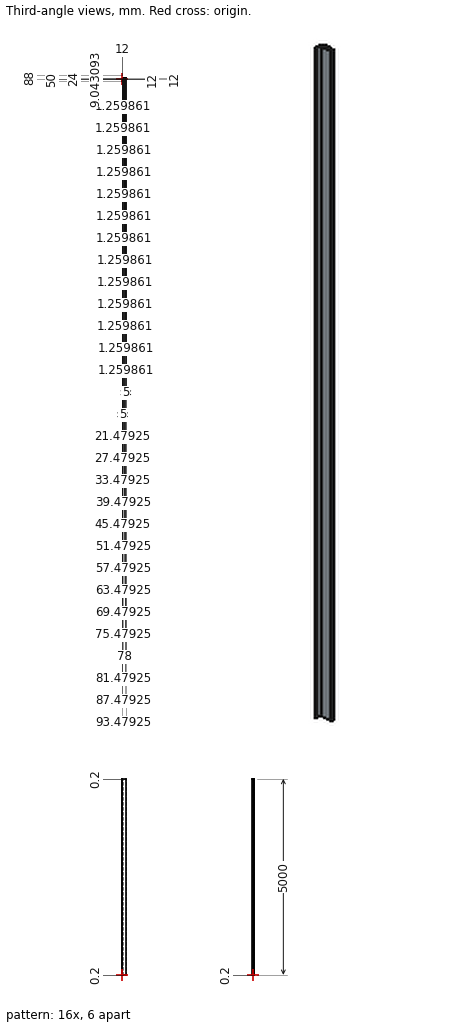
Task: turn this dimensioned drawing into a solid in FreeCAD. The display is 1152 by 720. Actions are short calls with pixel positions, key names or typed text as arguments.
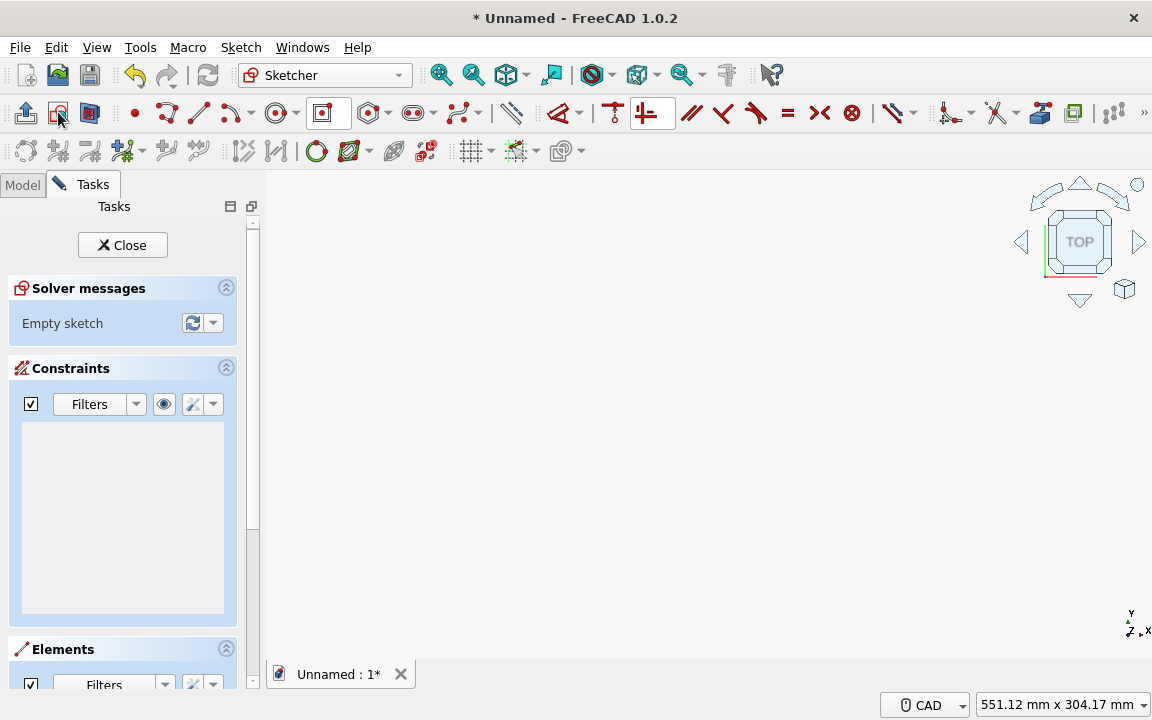
scroll(640, 414, down, 5)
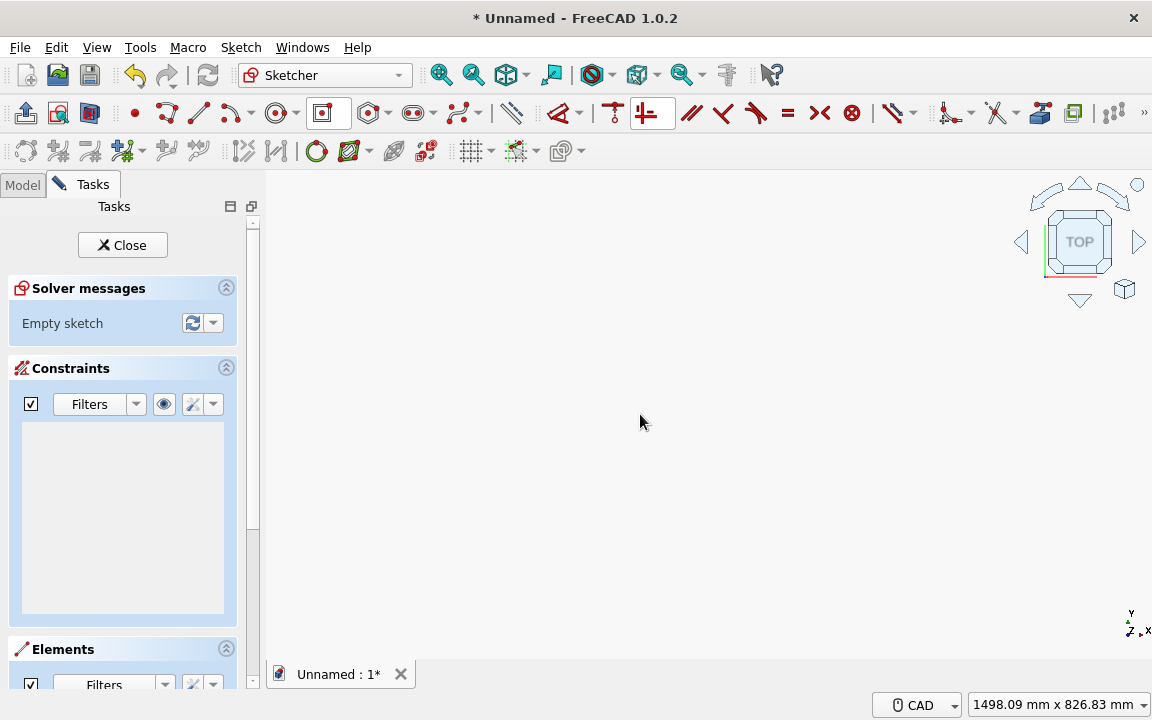
scroll(640, 414, down, 5)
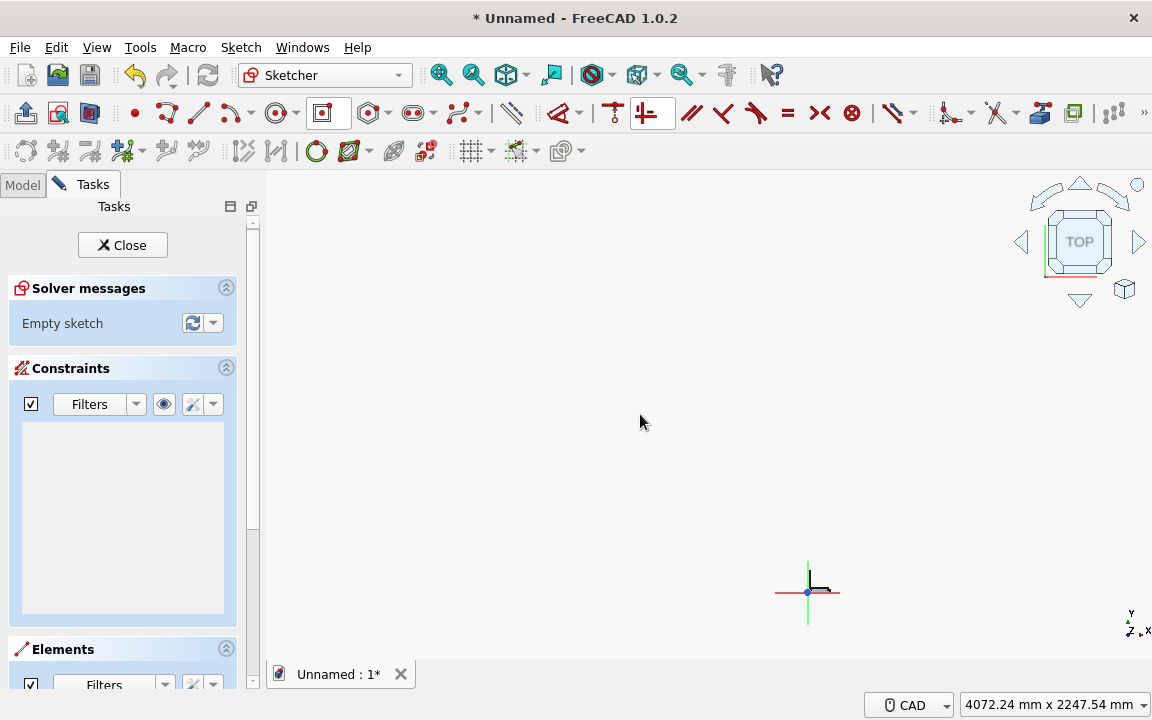
scroll(822, 598, up, 15)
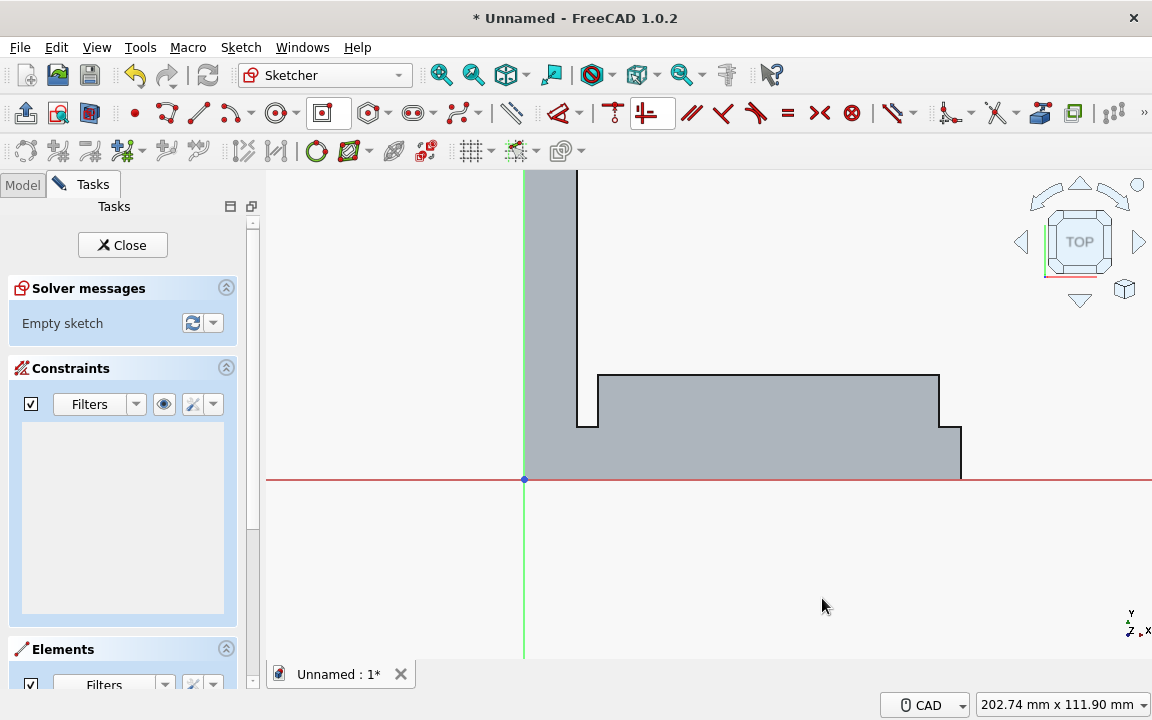
scroll(618, 392, up, 10)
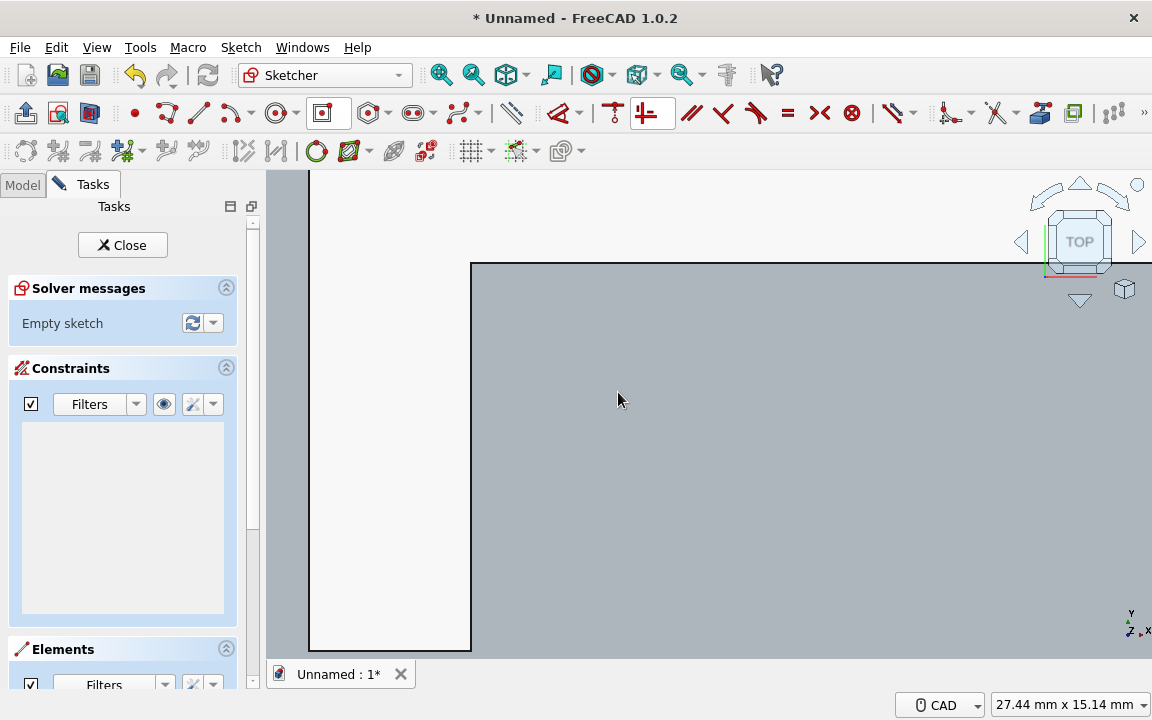
click(346, 114)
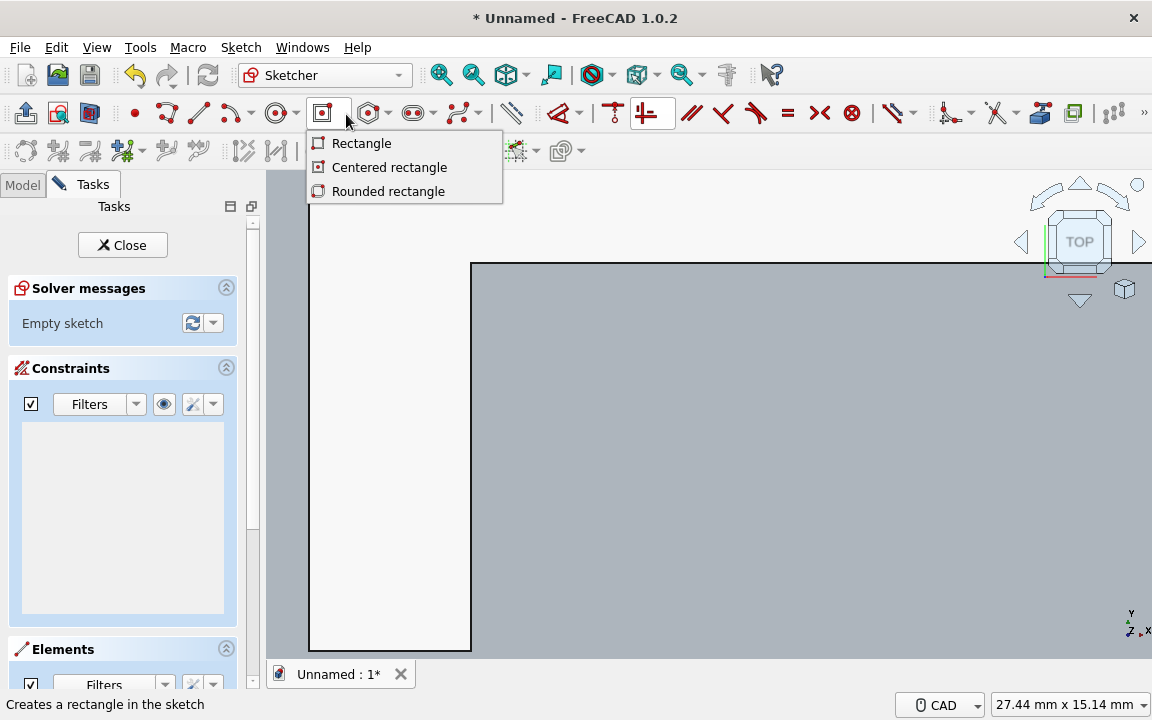
click(404, 143)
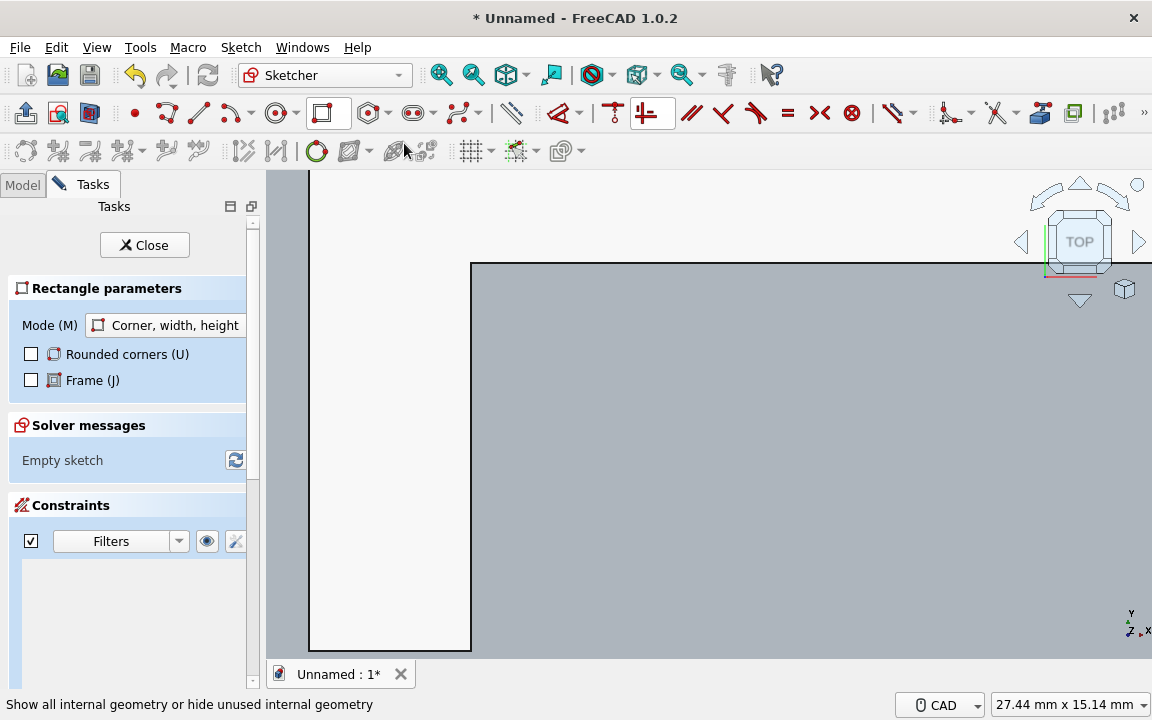
click(615, 263)
click(656, 555)
key(Escape)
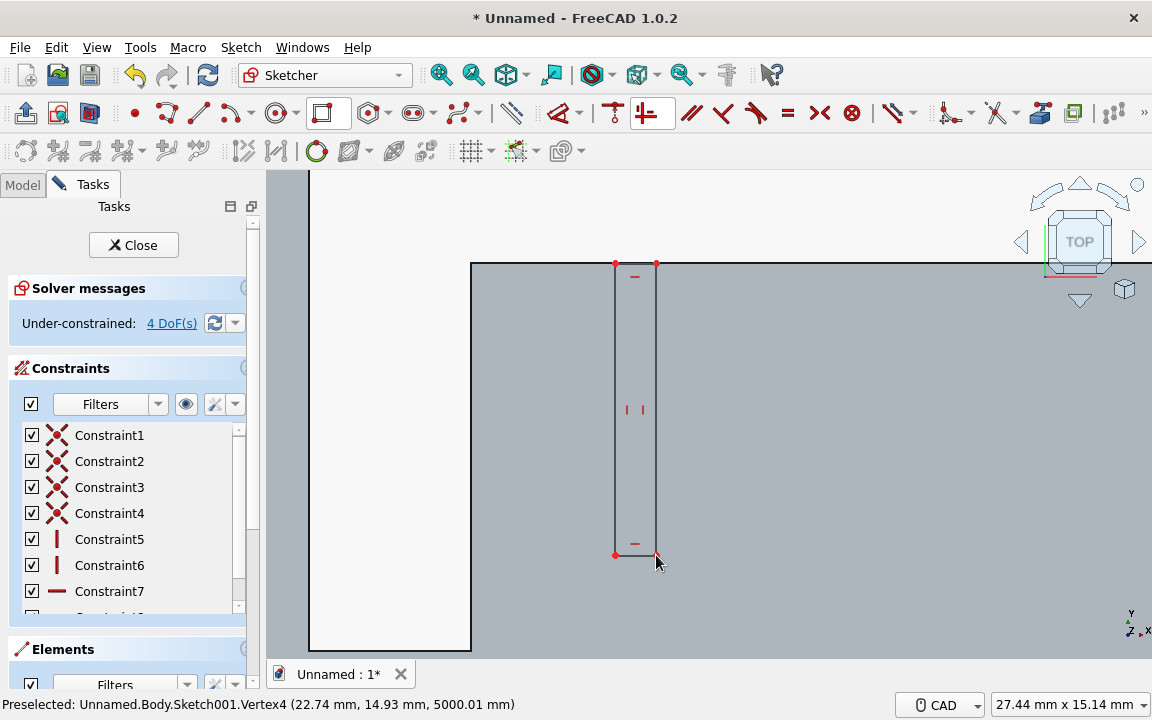
click(558, 114)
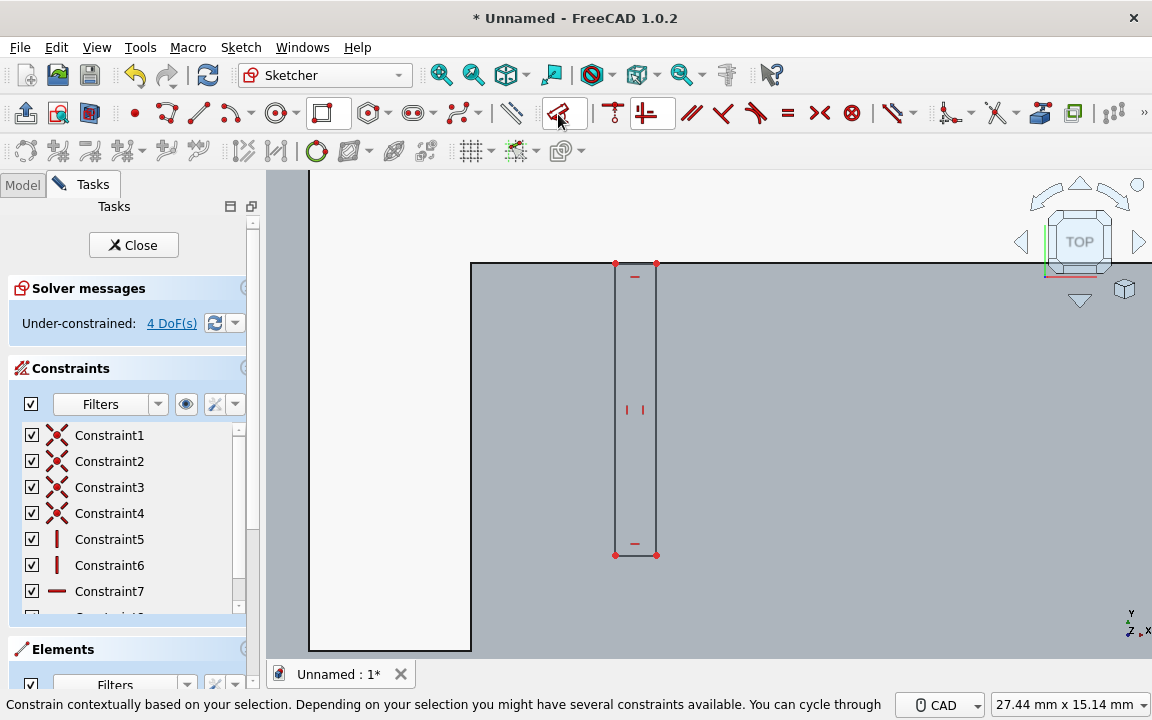
click(615, 264)
click(649, 576)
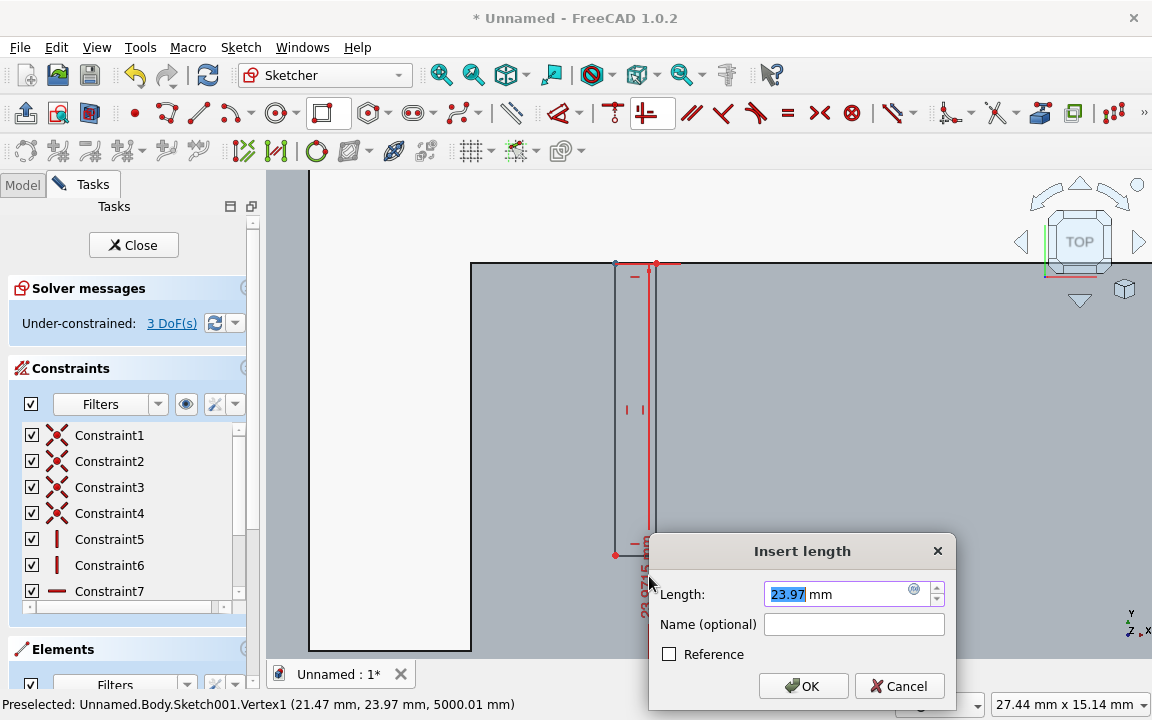
text(24)
key(Return)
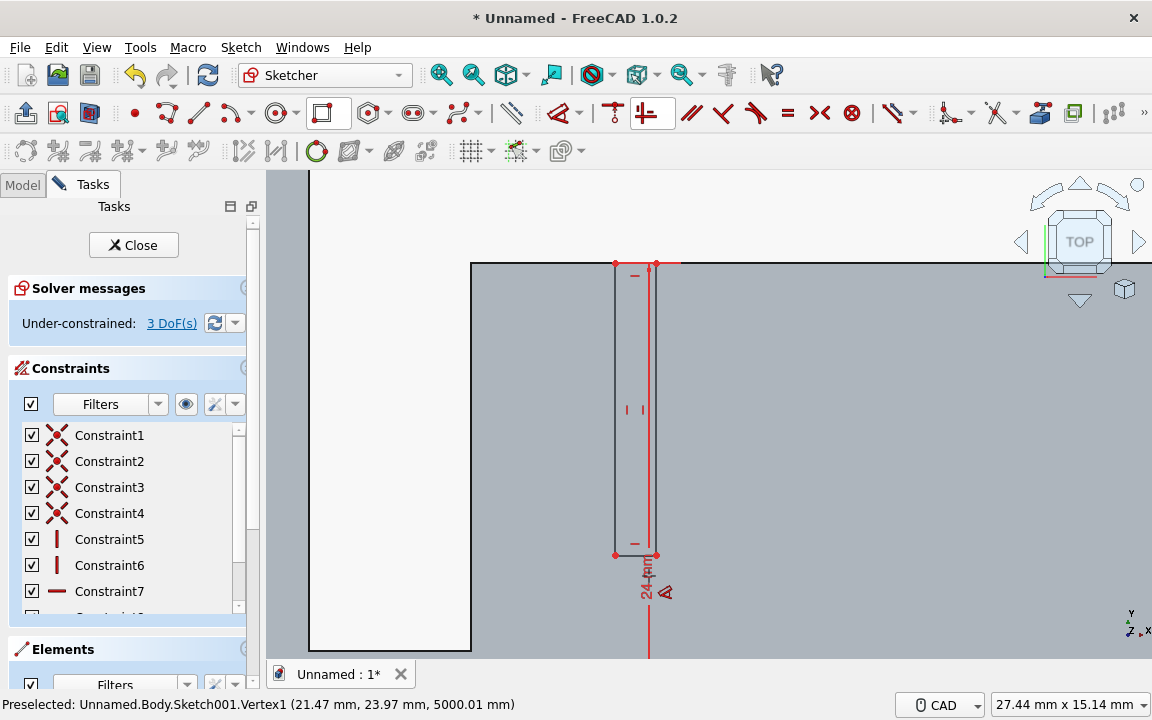
click(615, 351)
click(581, 410)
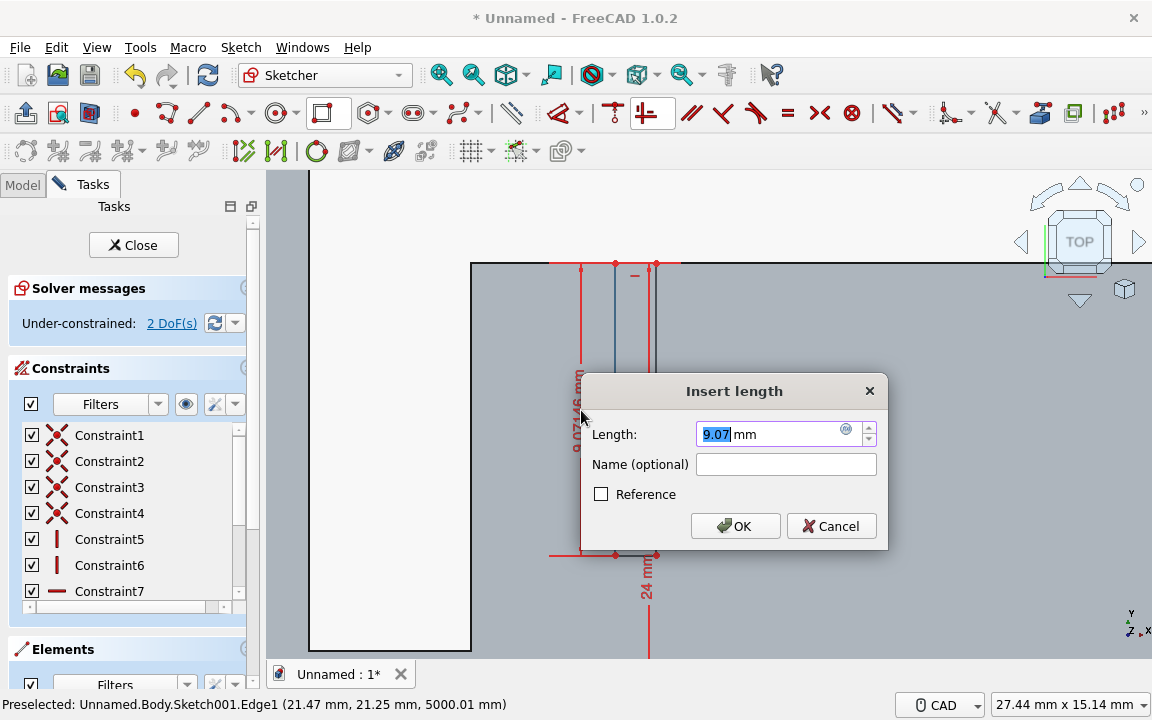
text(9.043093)
key(Return)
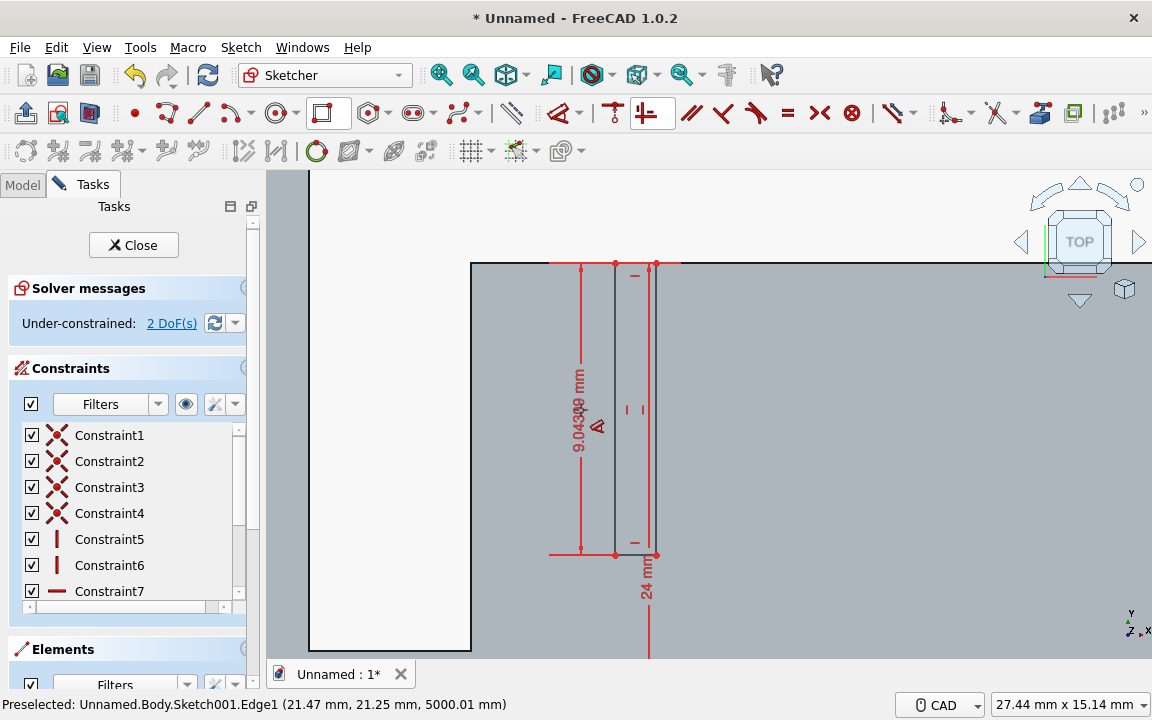
click(627, 555)
click(636, 521)